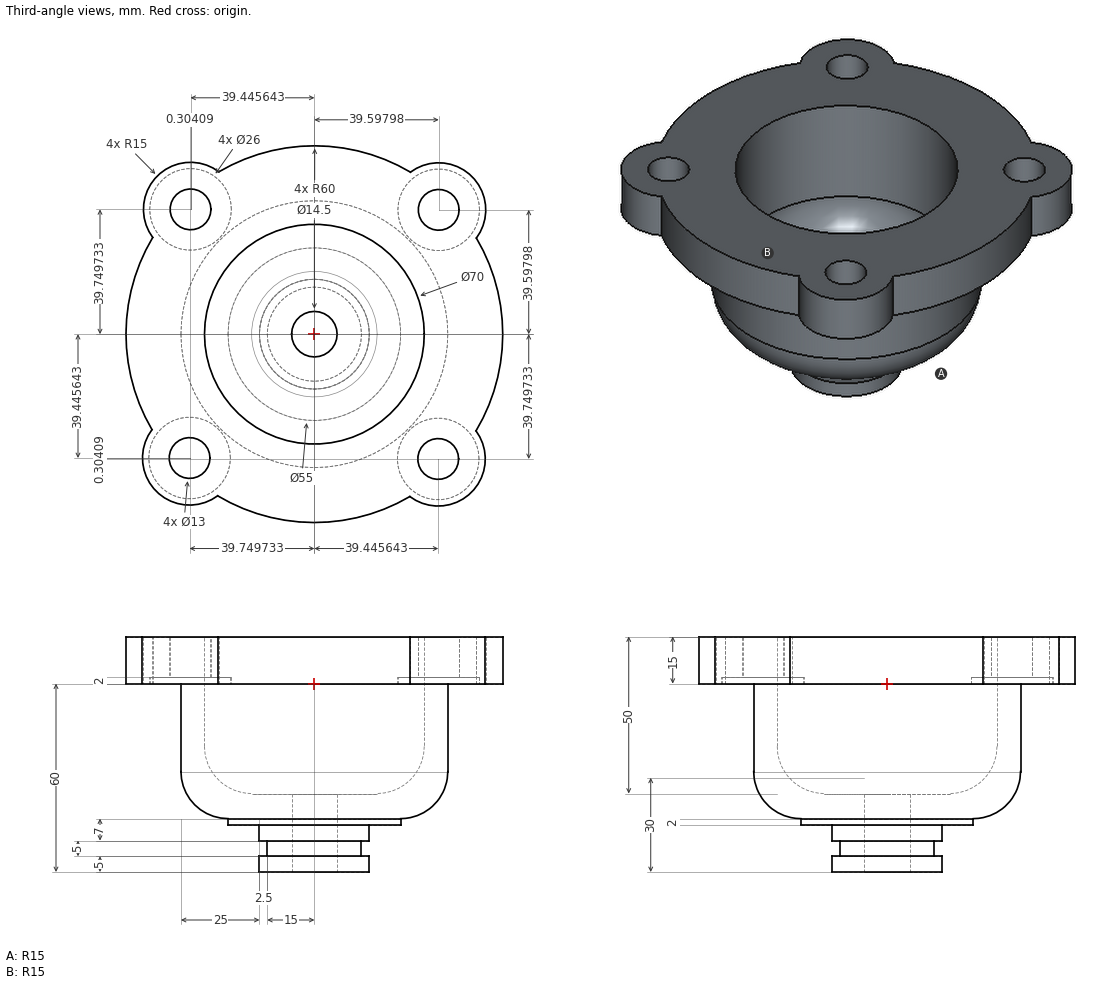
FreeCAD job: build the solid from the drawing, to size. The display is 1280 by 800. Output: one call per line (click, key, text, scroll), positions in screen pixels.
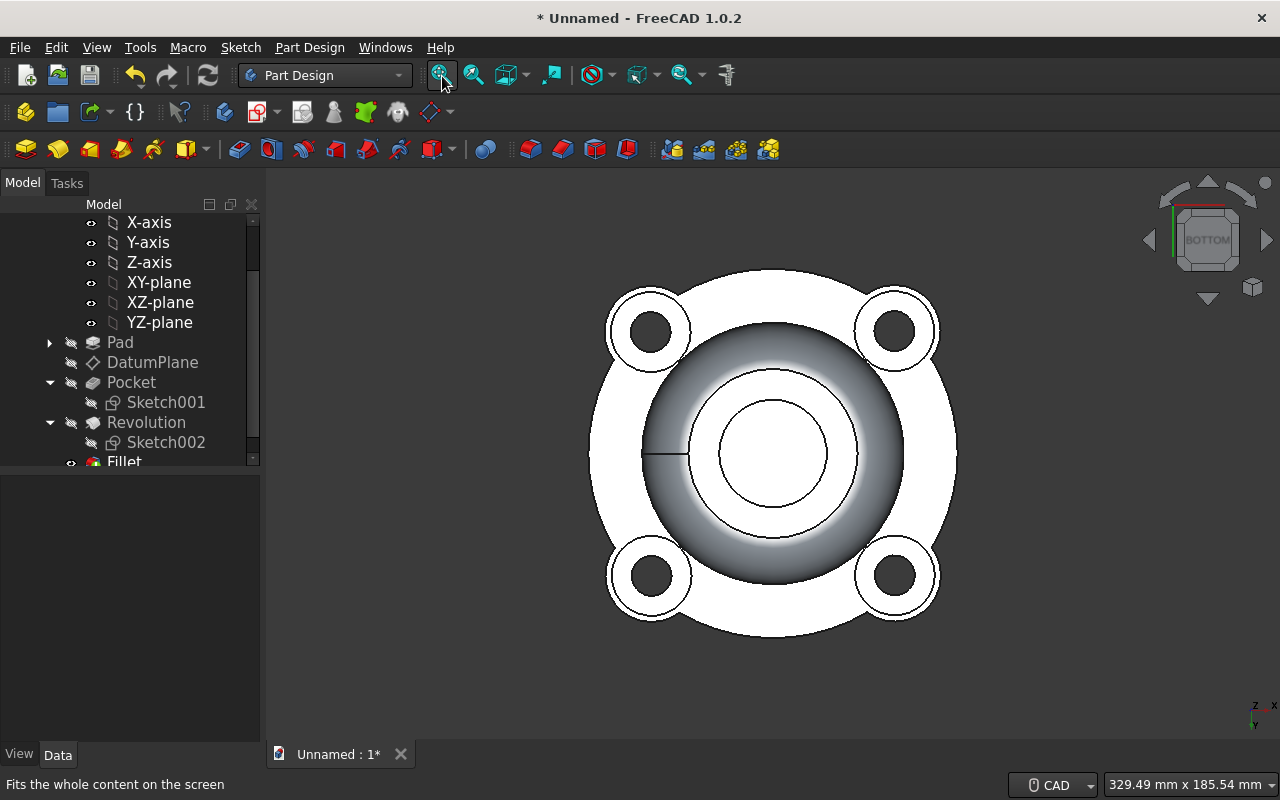
click(821, 404)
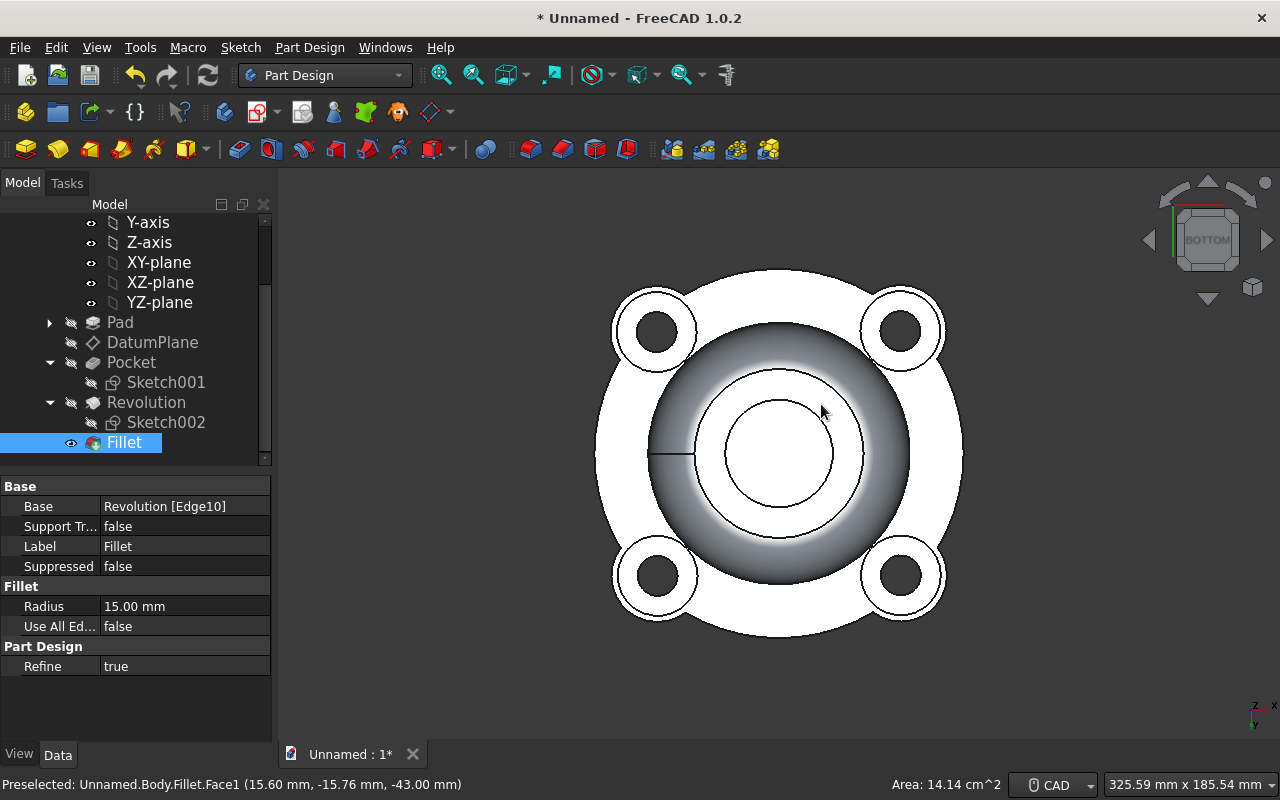
click(258, 112)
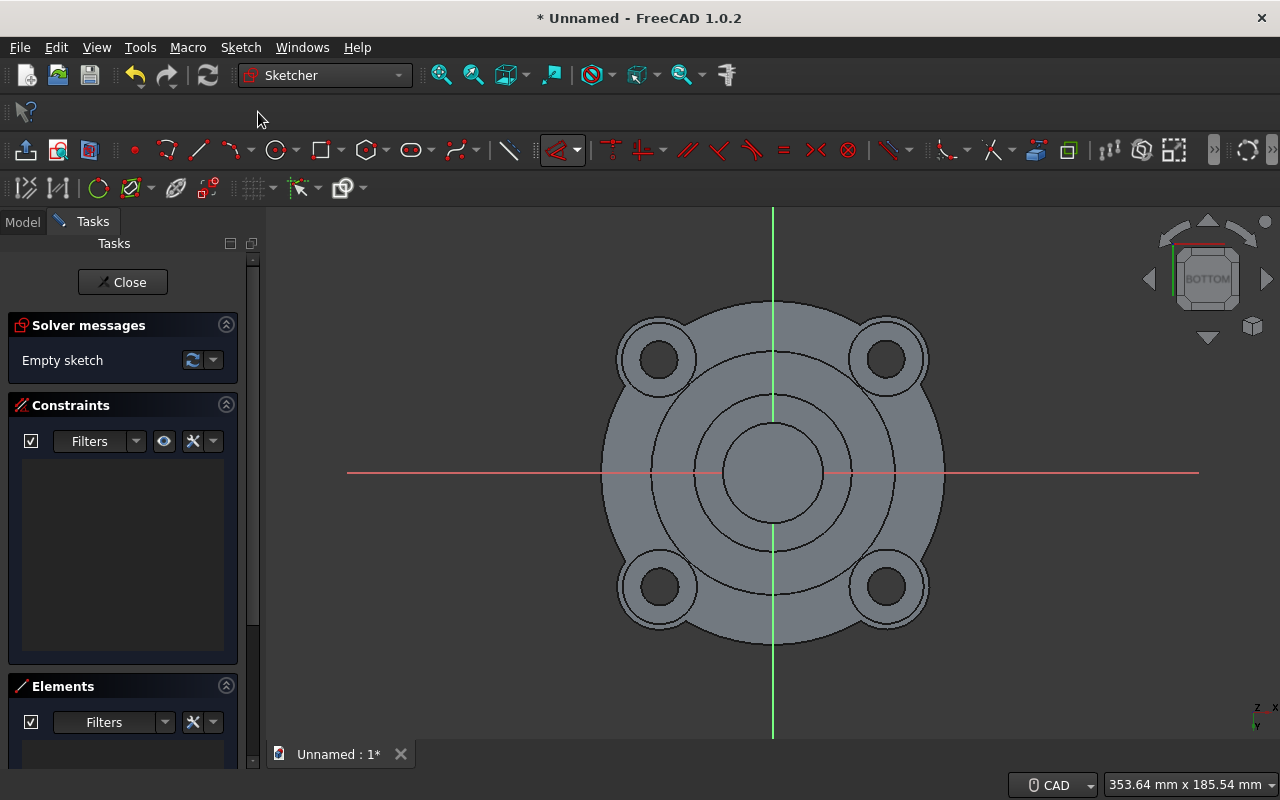
scroll(829, 473, up, 4)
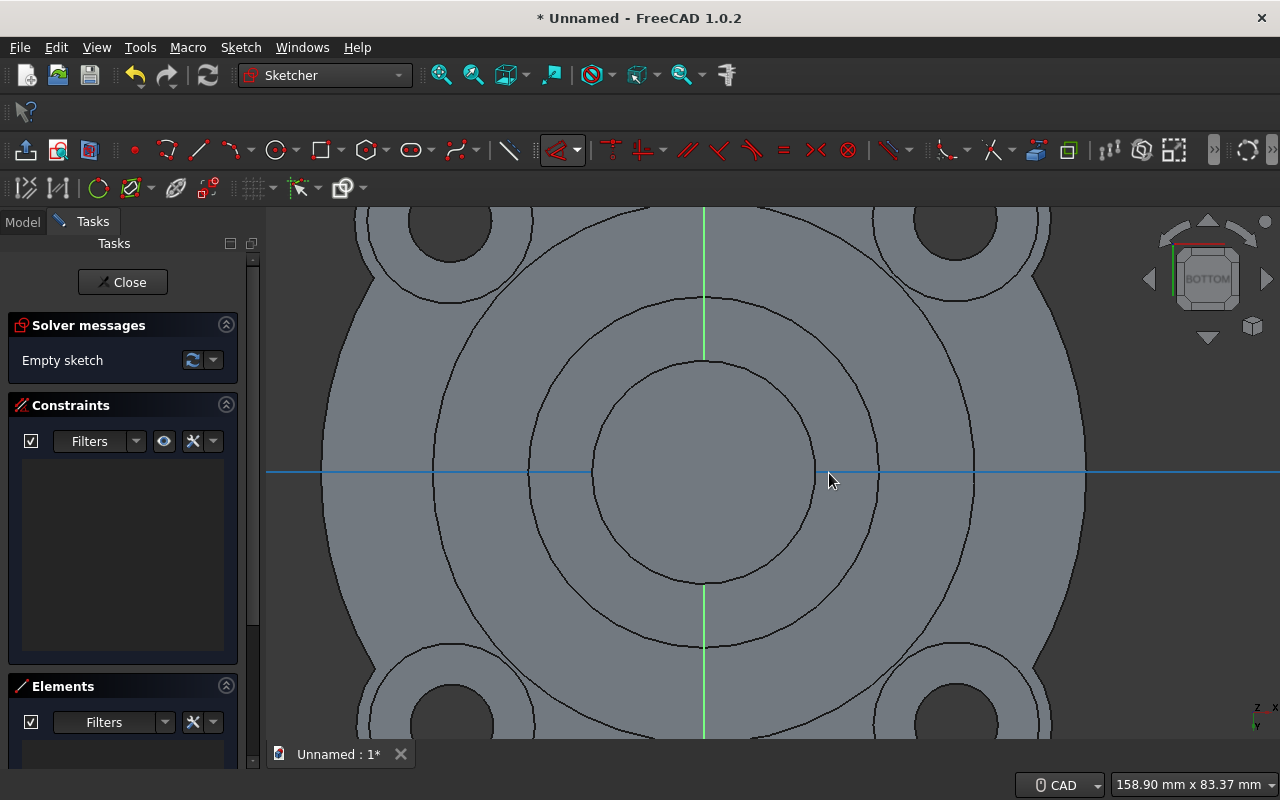
click(276, 150)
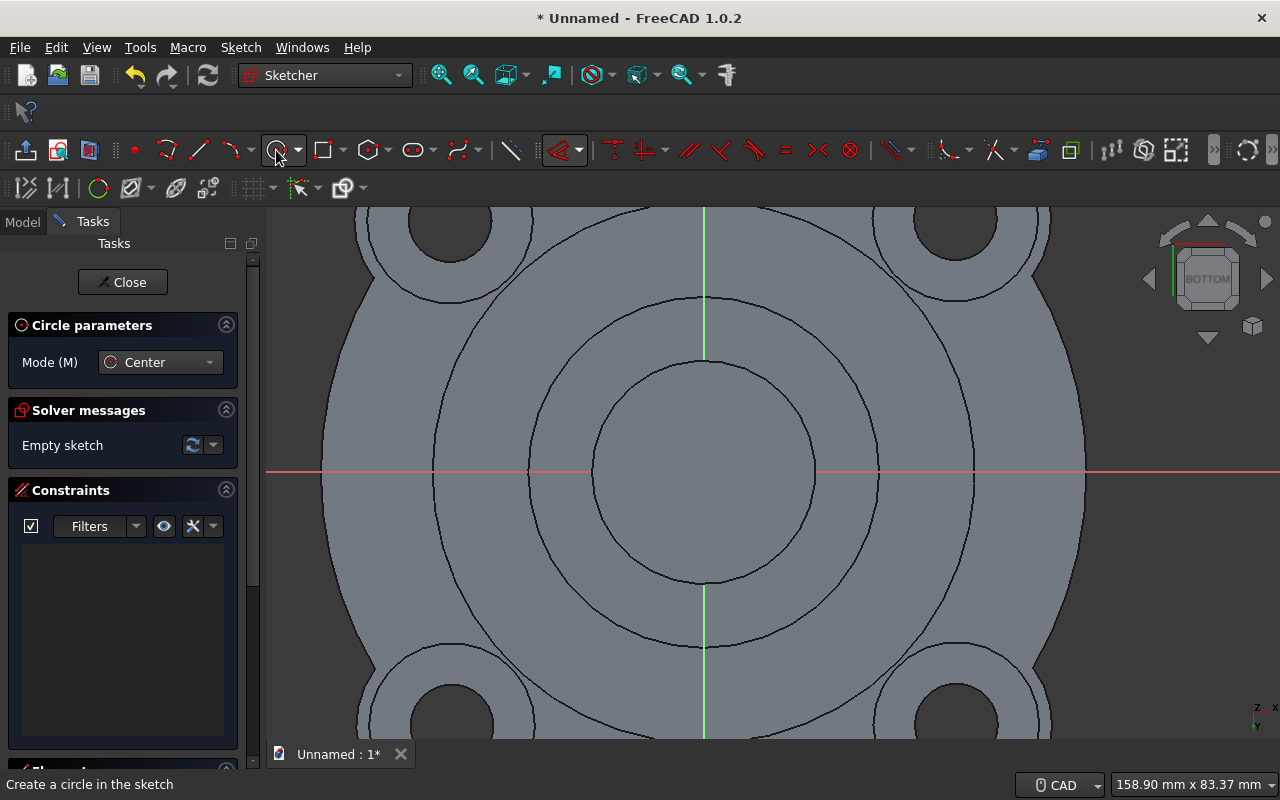
click(704, 472)
move(828, 348)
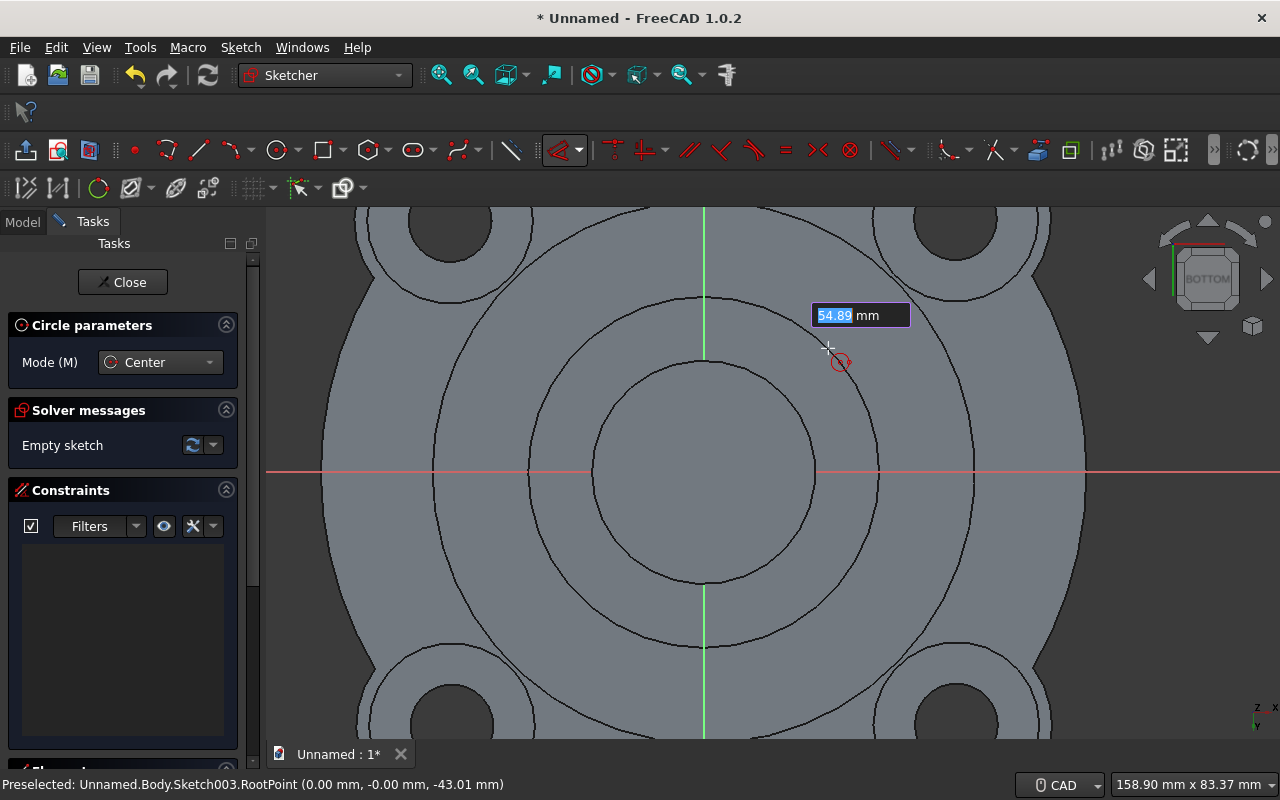
text(55)
key(Return)
key(Escape)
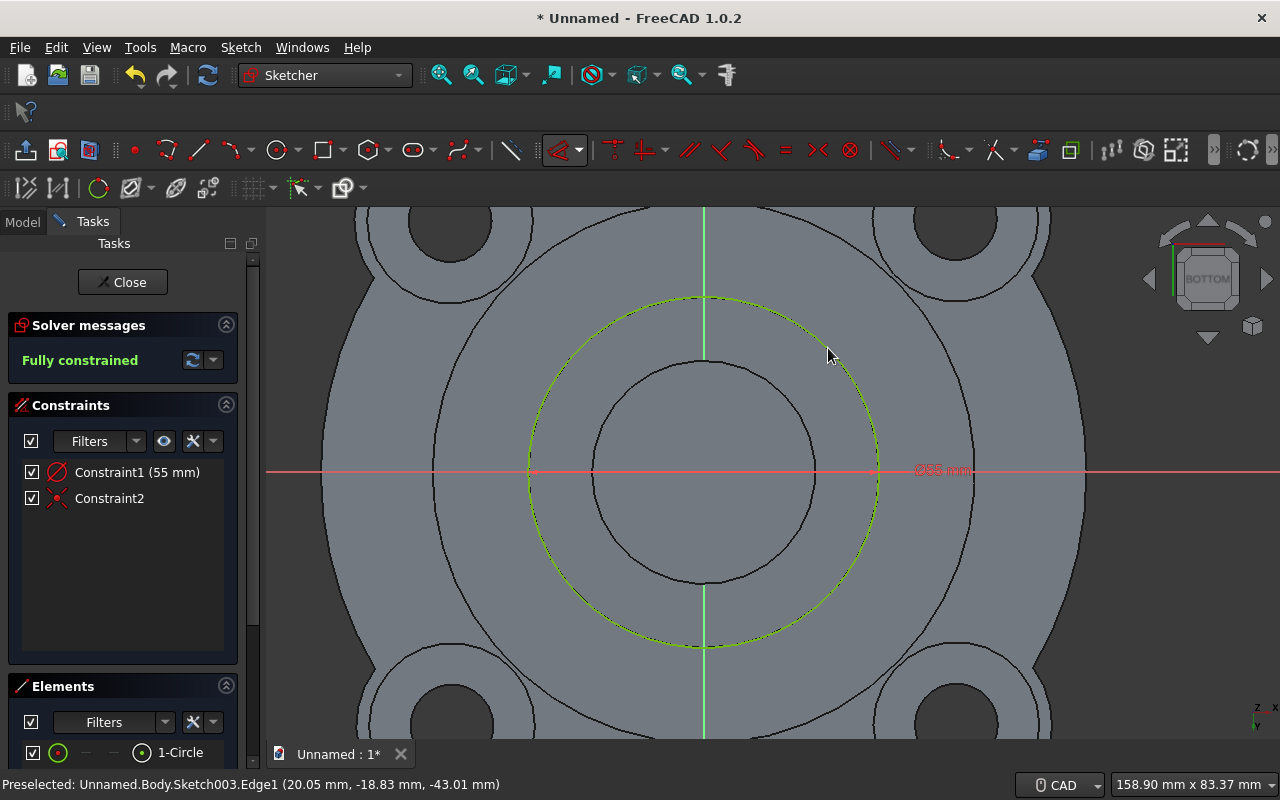
click(123, 282)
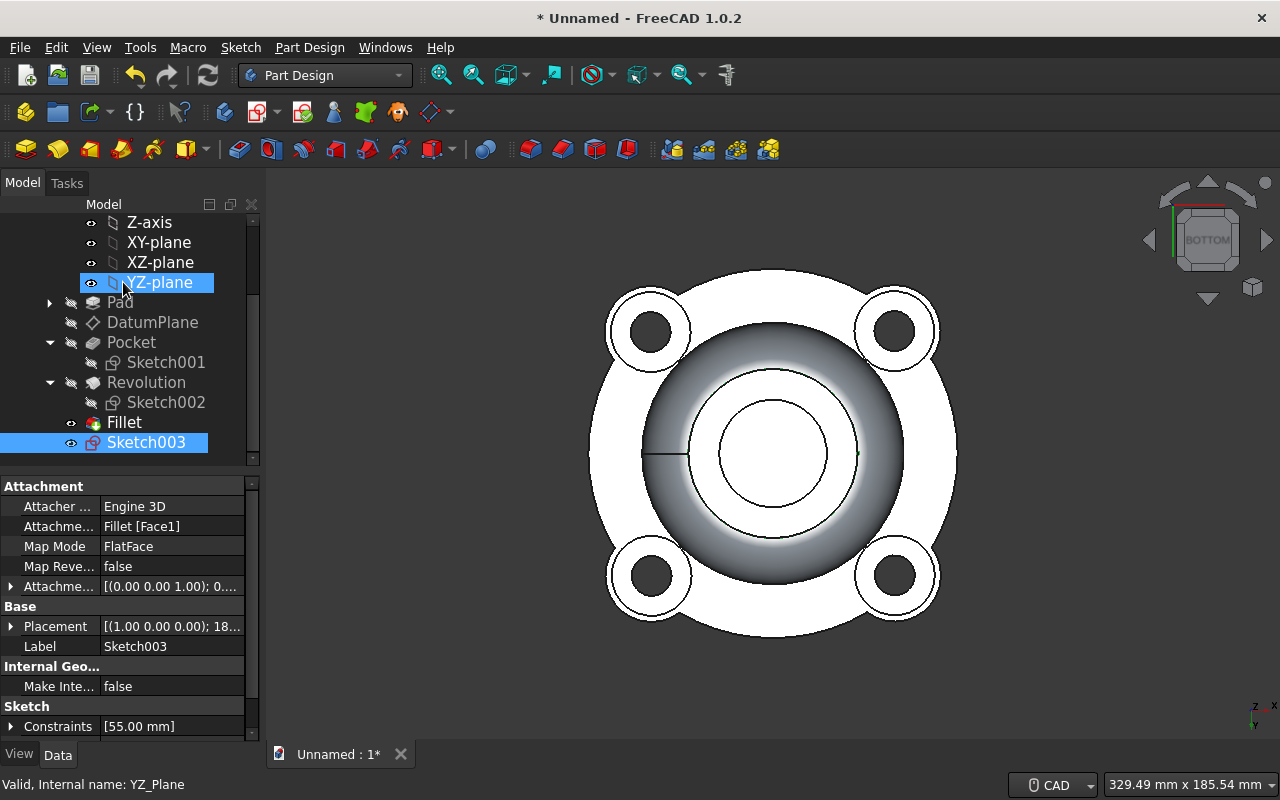
click(26, 150)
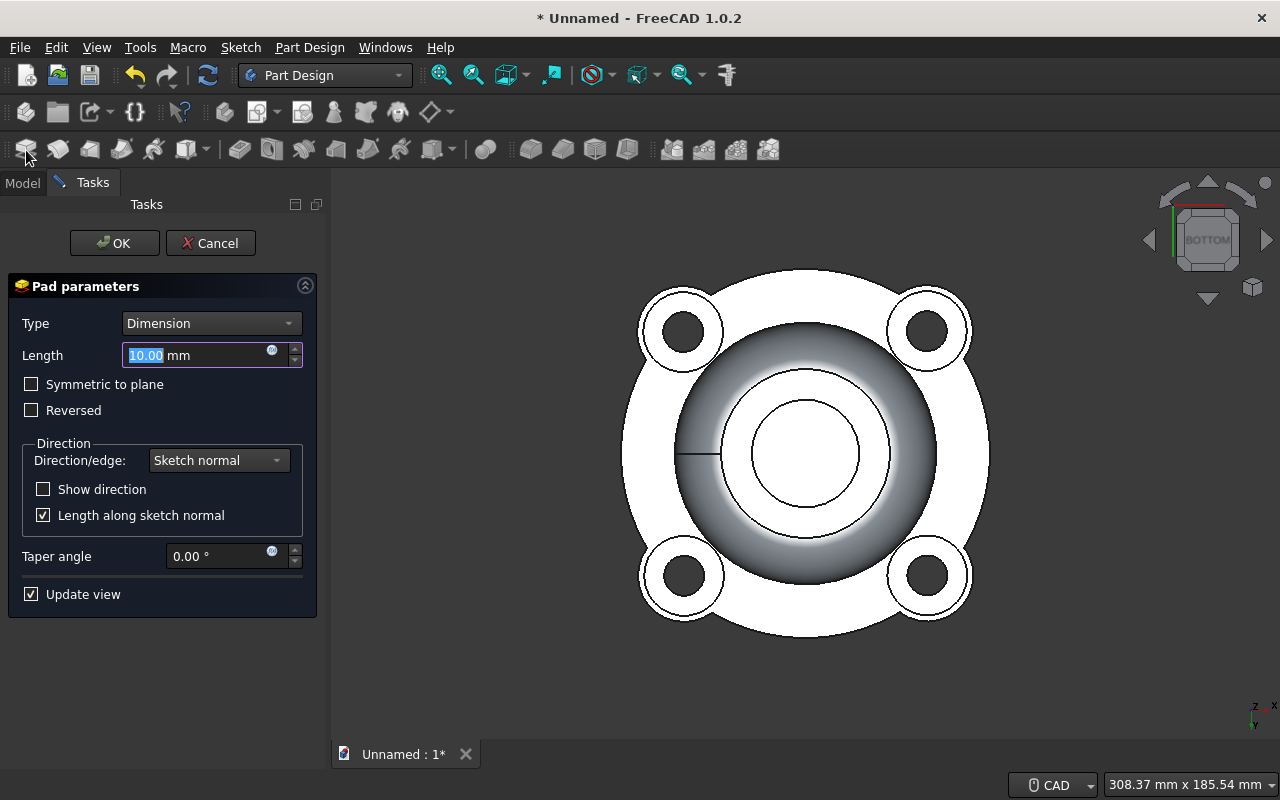
text(2)
key(Tab)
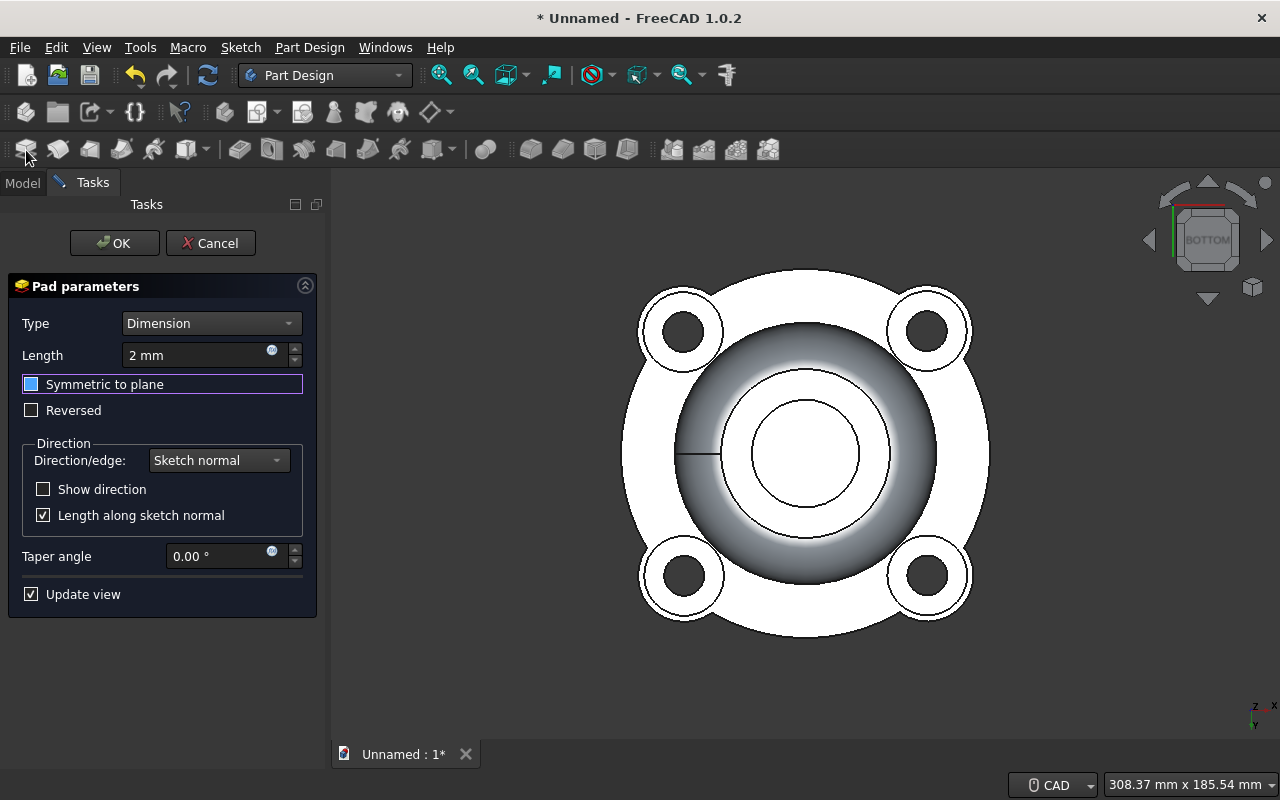
click(115, 243)